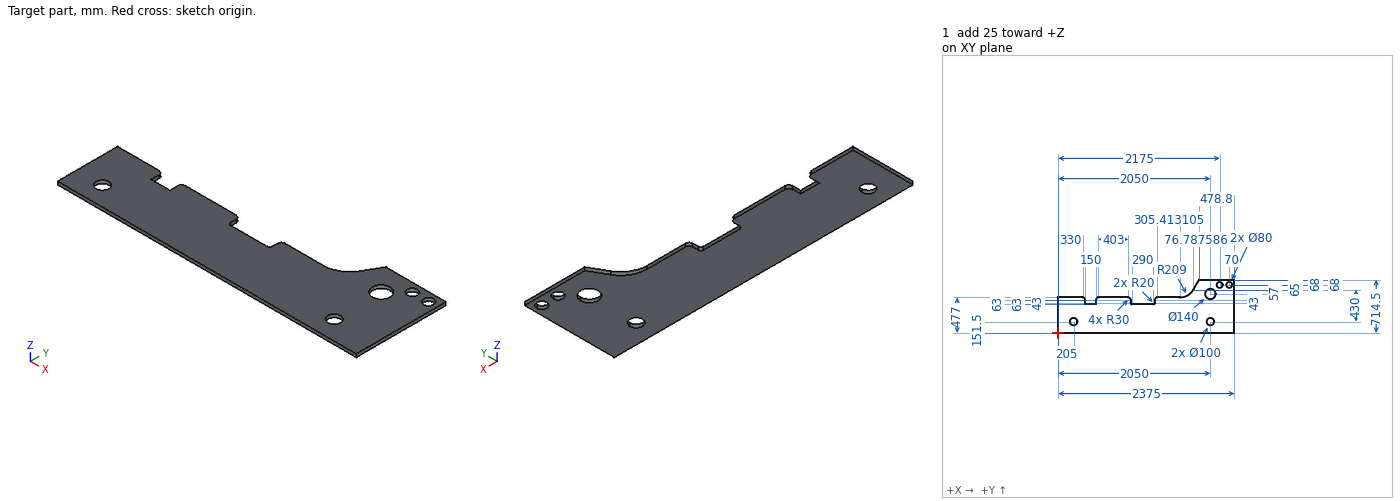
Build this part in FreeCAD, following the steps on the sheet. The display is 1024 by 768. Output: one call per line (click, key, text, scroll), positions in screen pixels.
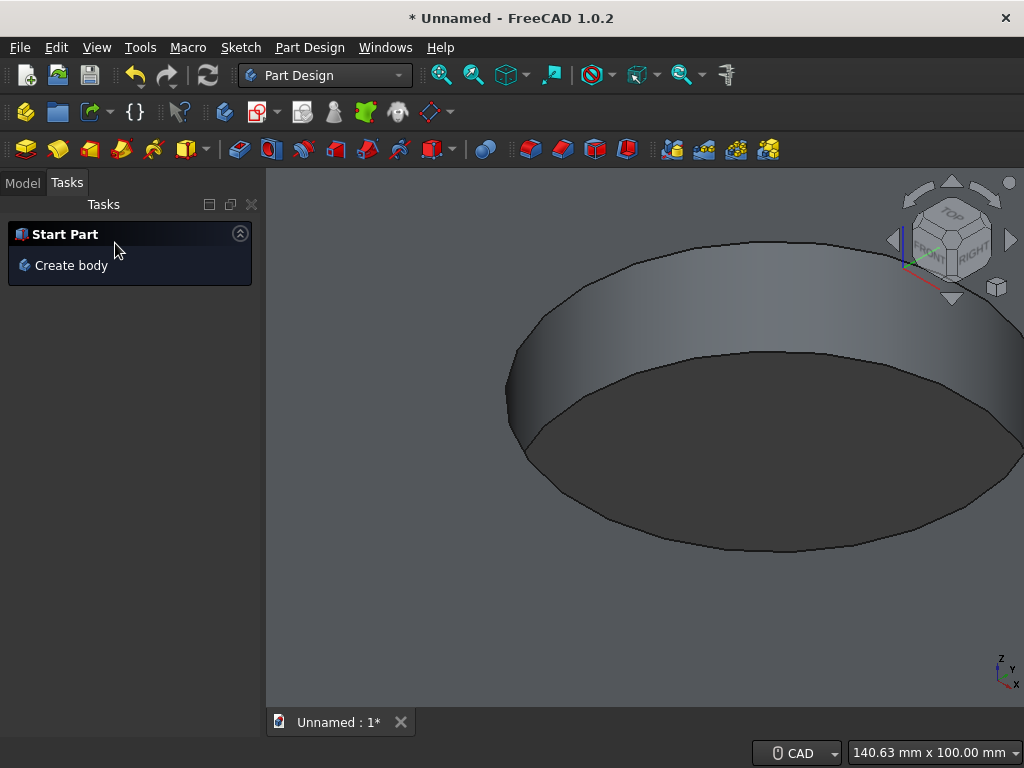
click(442, 76)